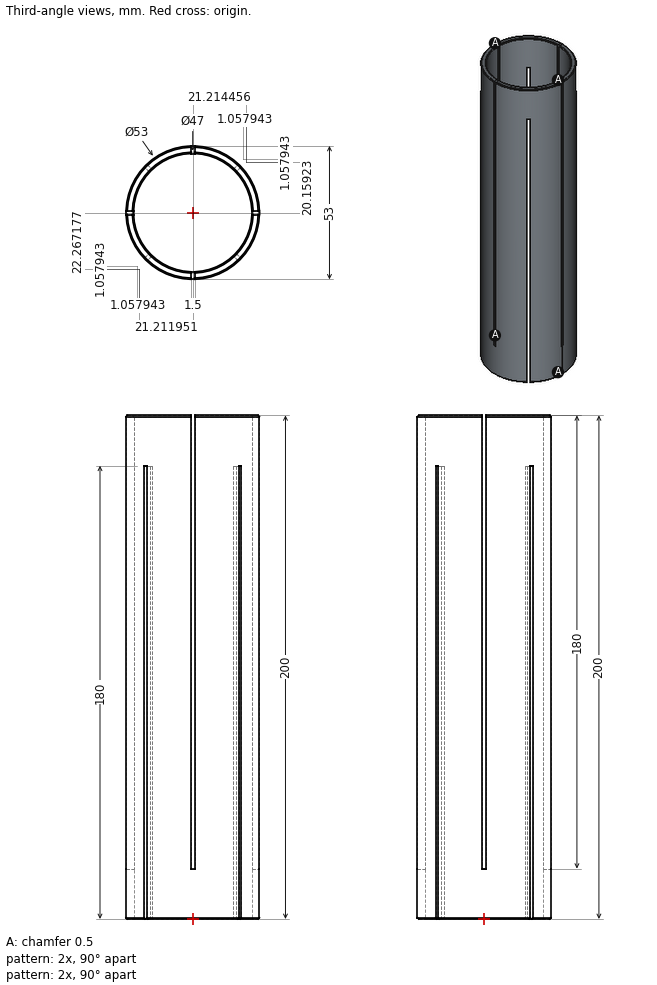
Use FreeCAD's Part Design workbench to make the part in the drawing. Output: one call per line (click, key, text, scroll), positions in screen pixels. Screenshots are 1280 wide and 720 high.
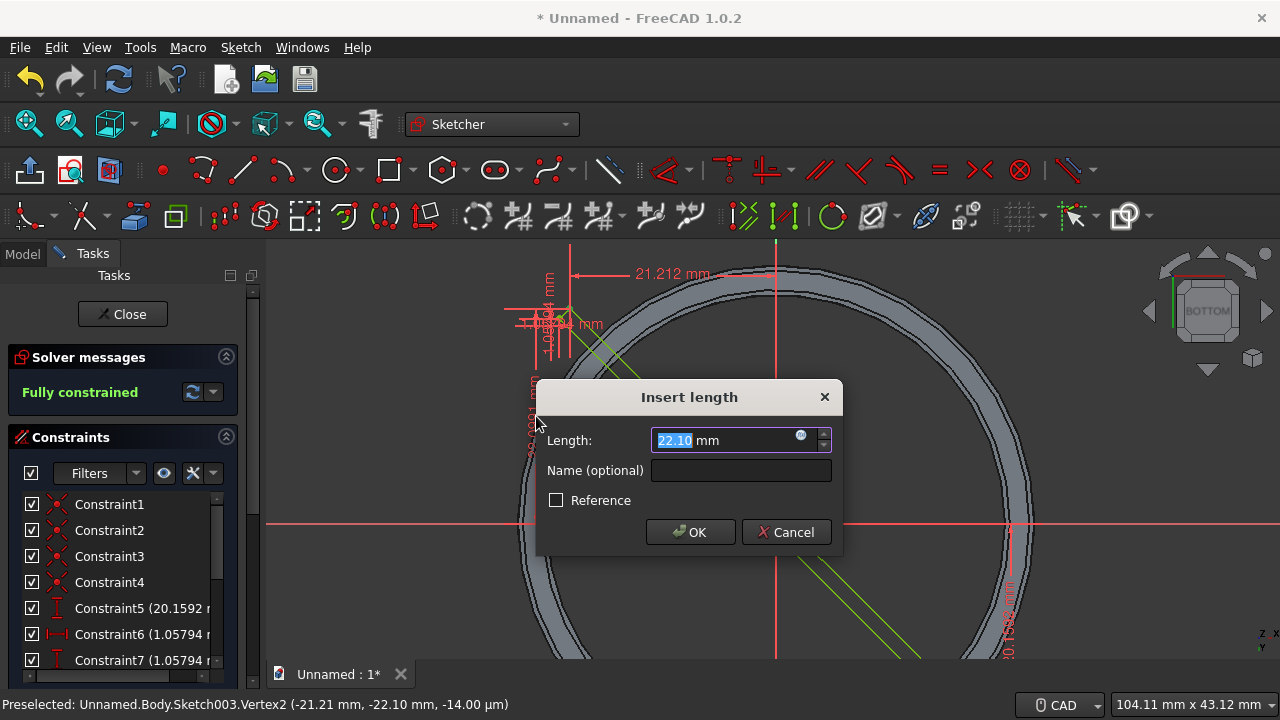
text(22.267177)
key(Return)
key(Escape)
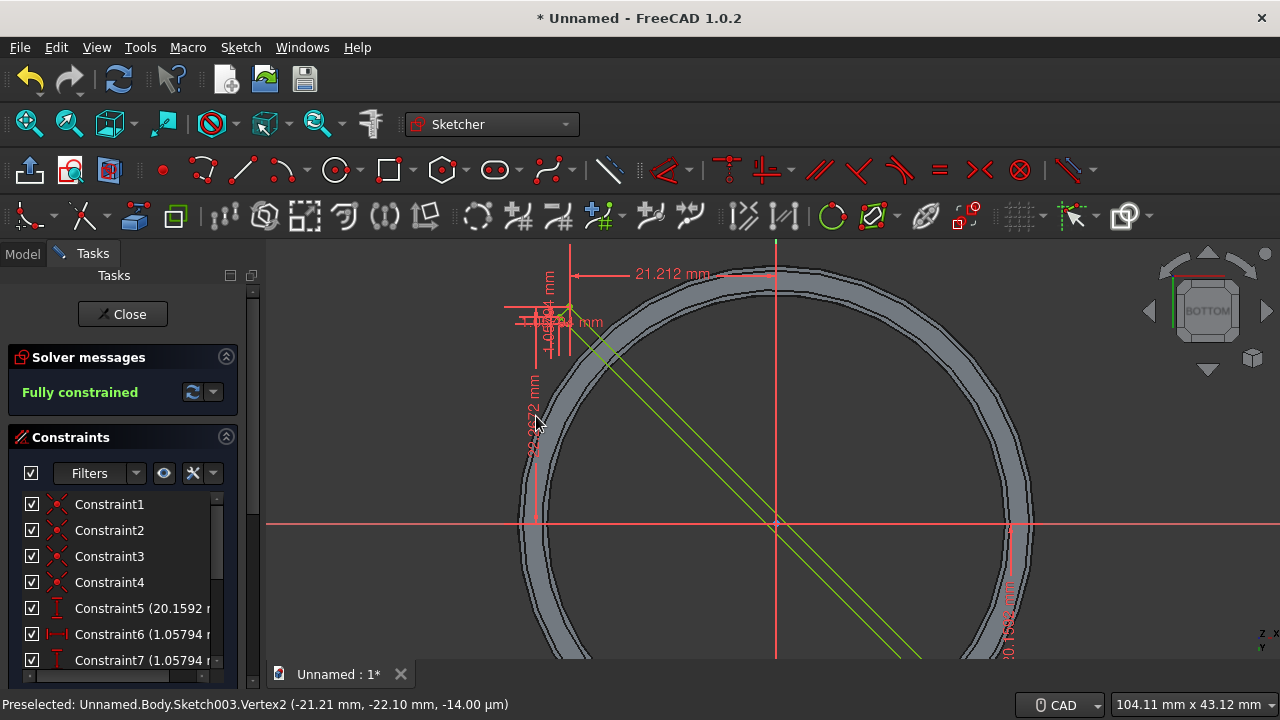
click(123, 314)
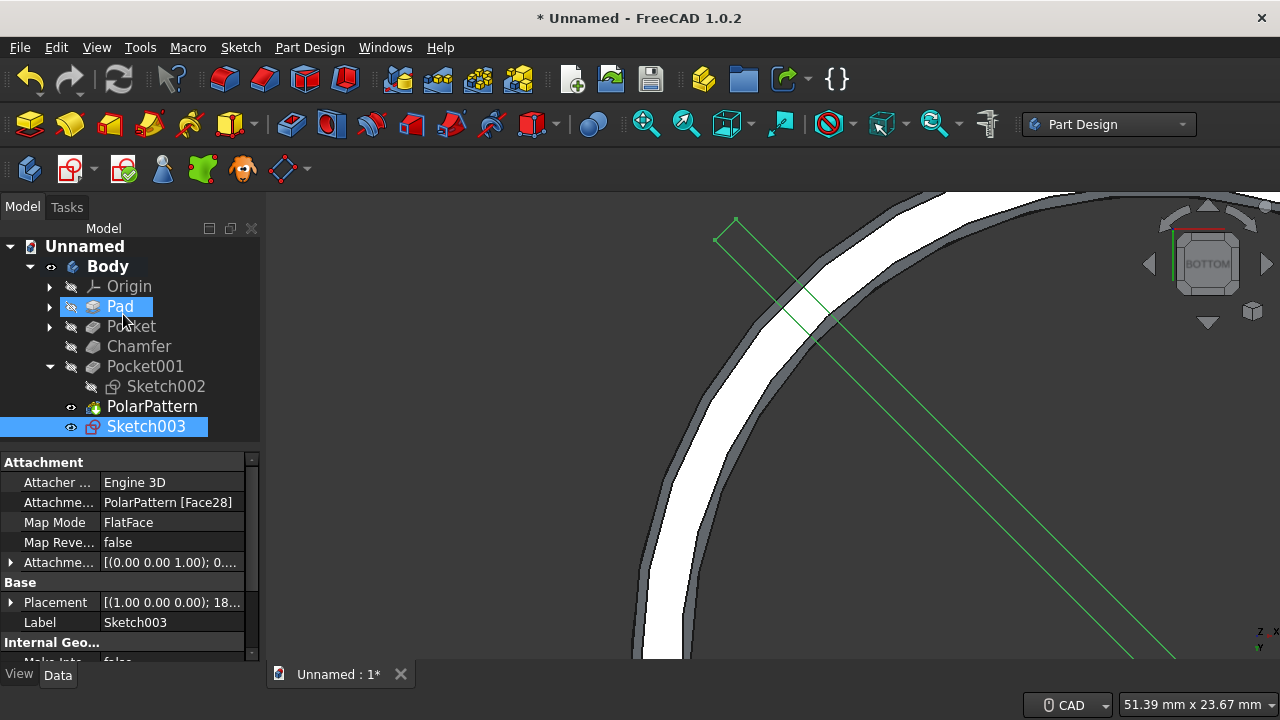
click(292, 124)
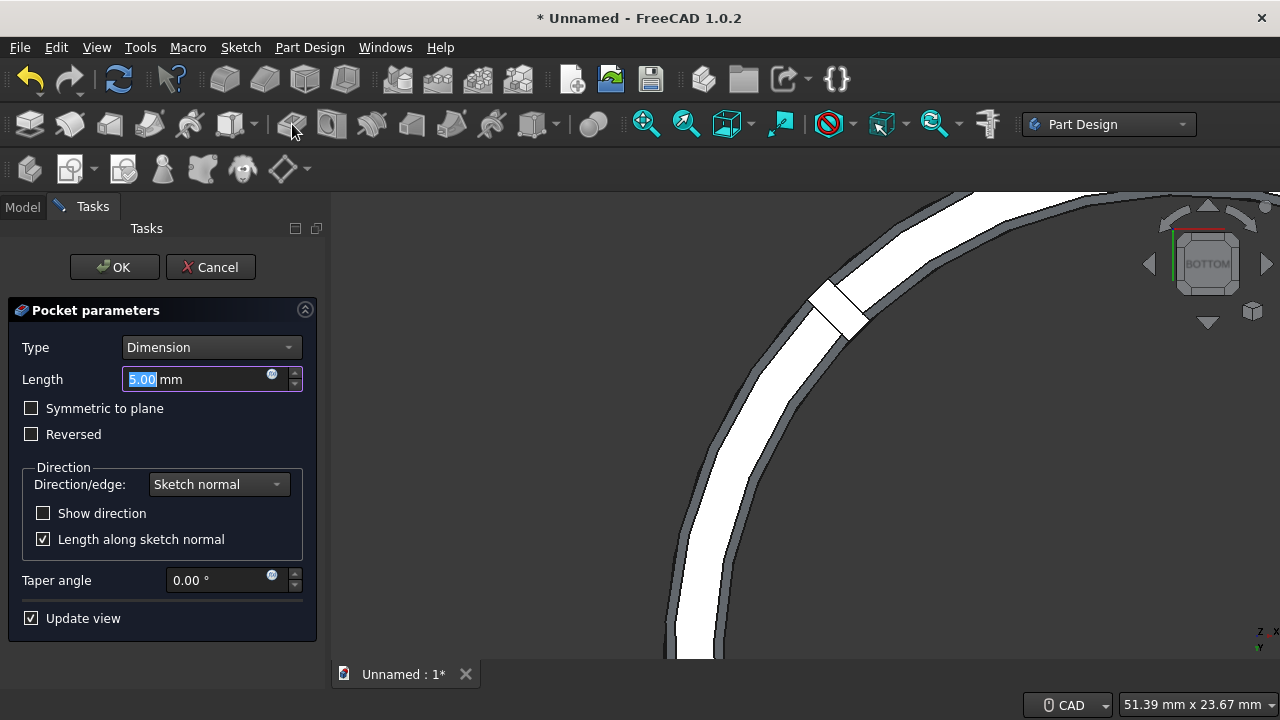
text(180)
key(Tab)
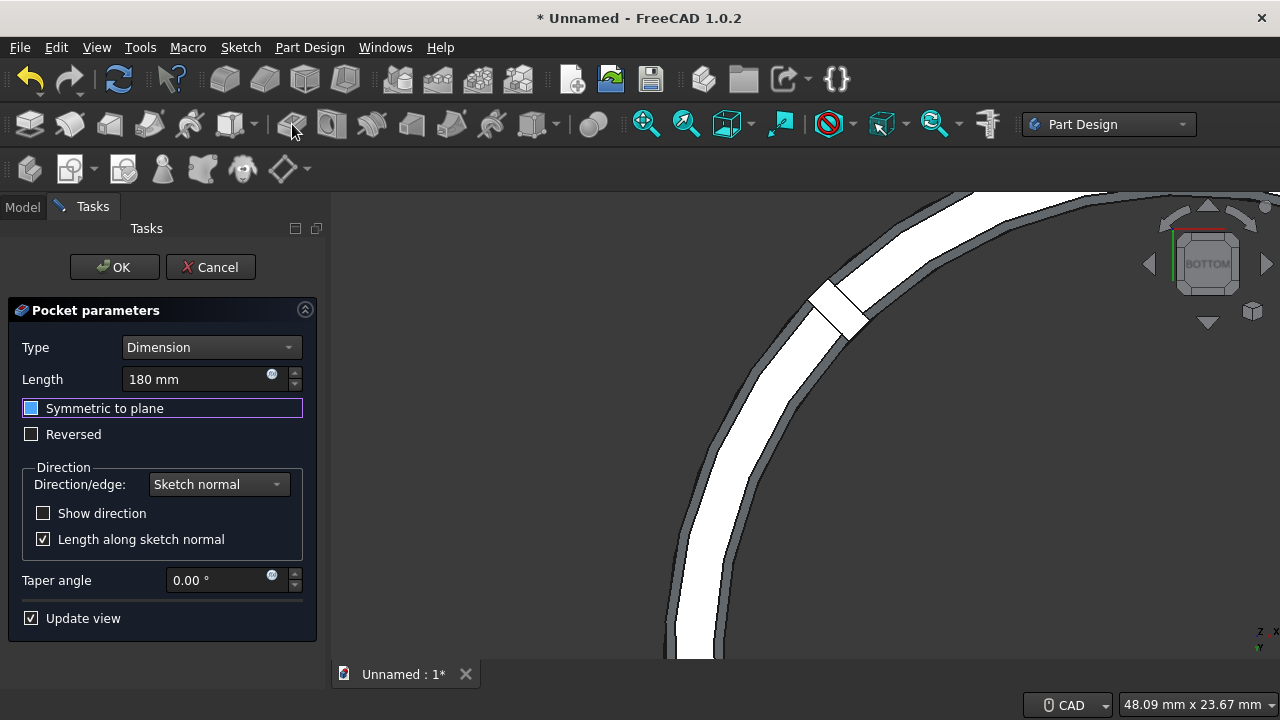
click(115, 267)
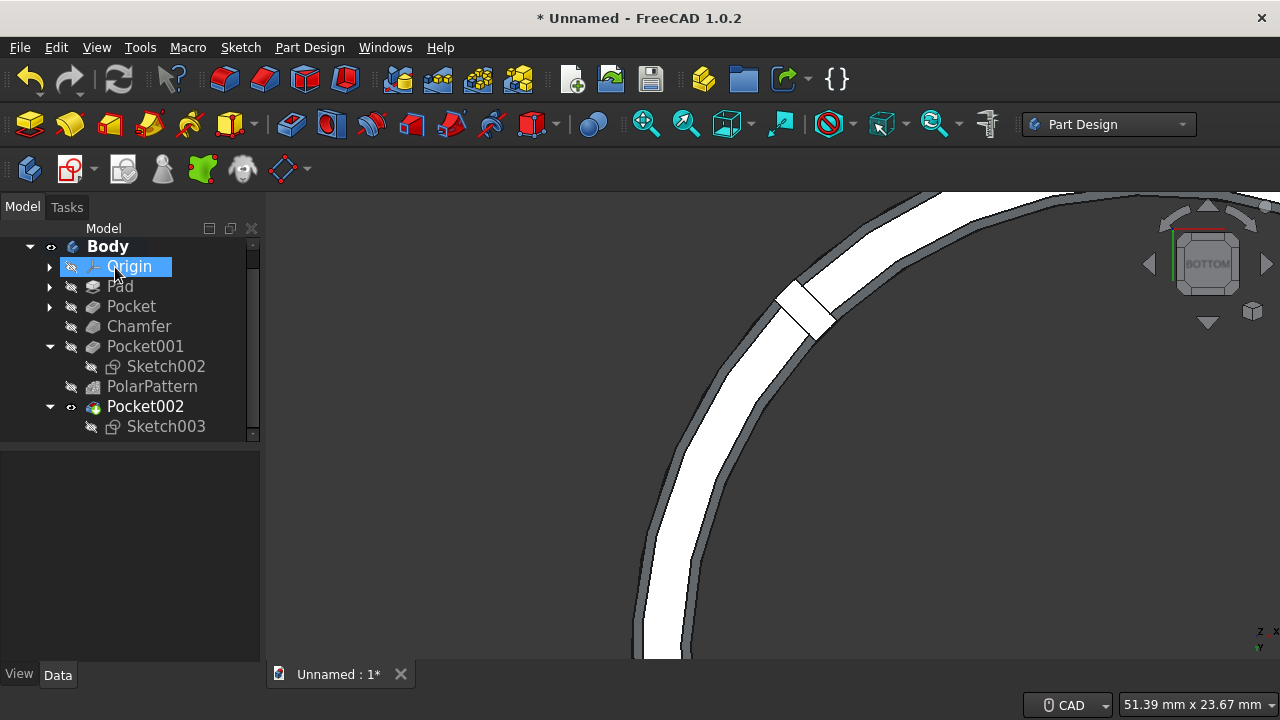
click(648, 124)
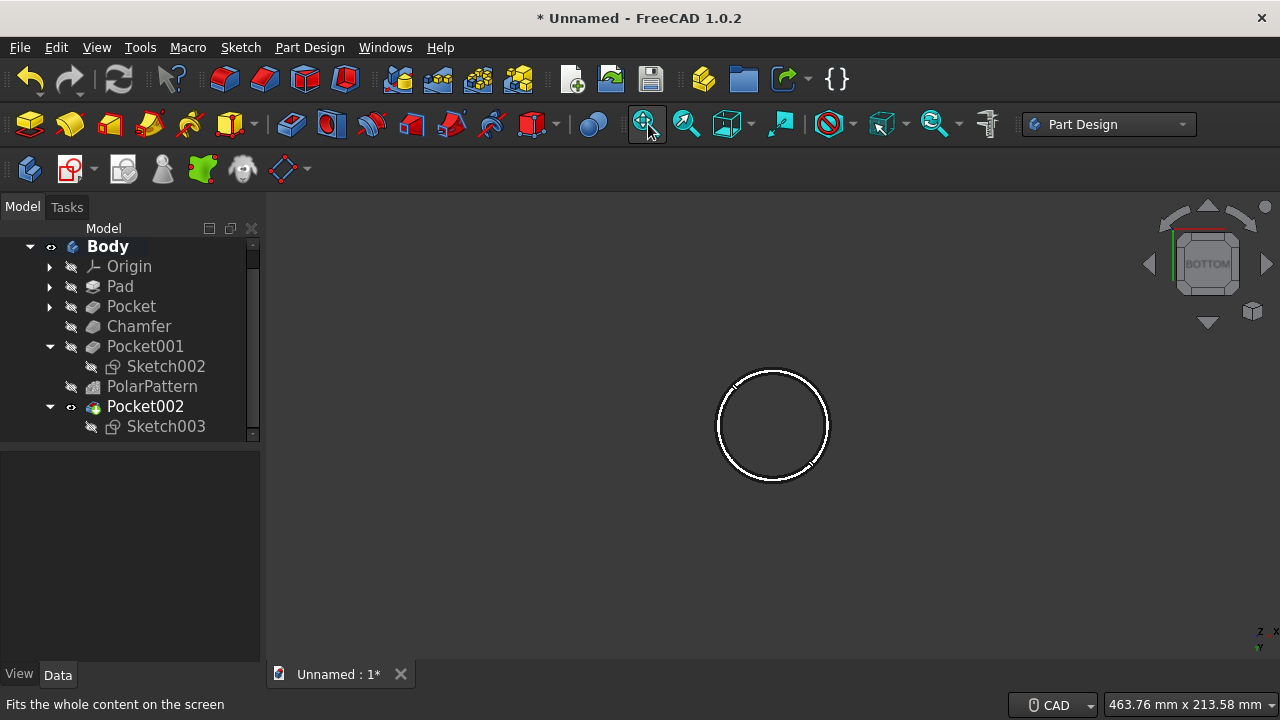
click(116, 407)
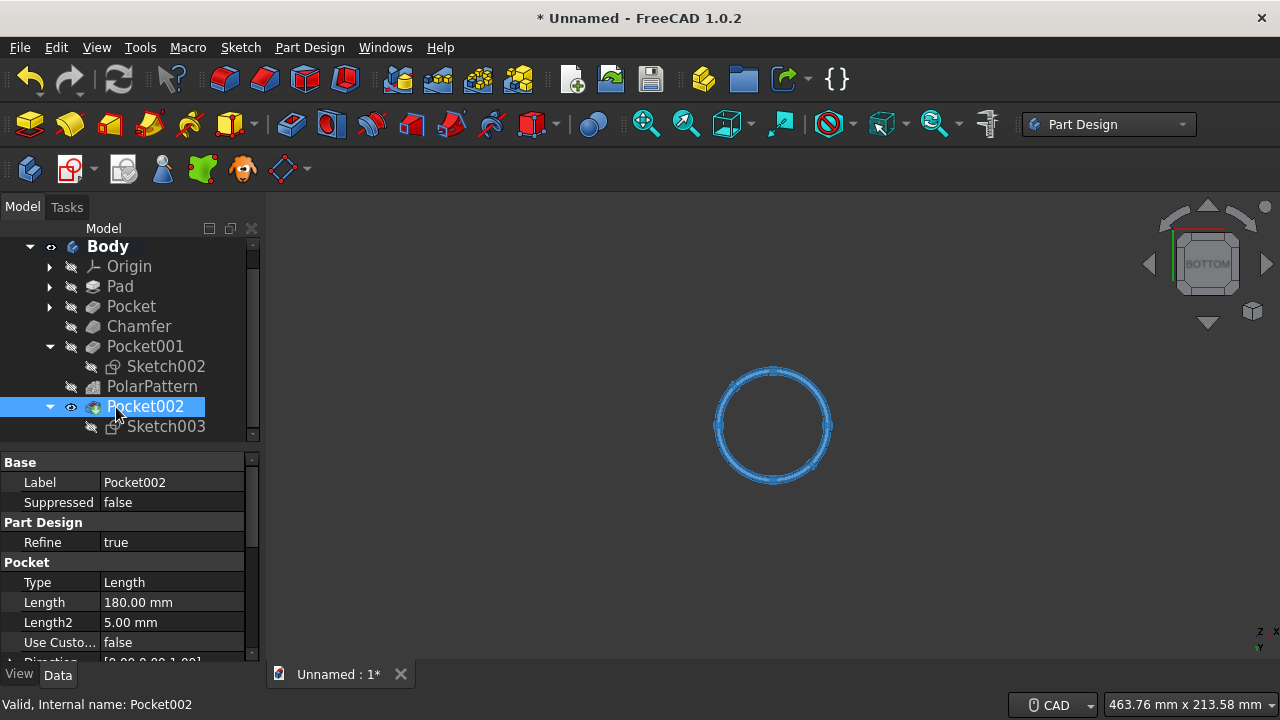
click(478, 80)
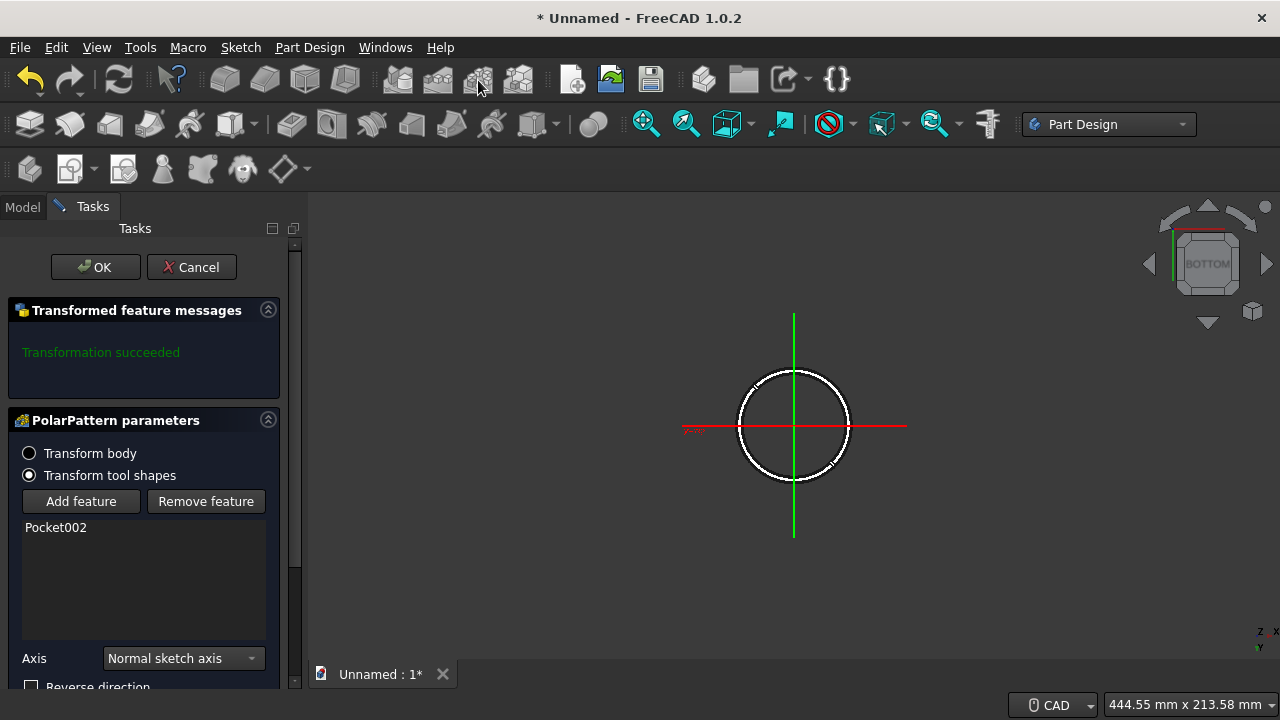
click(184, 658)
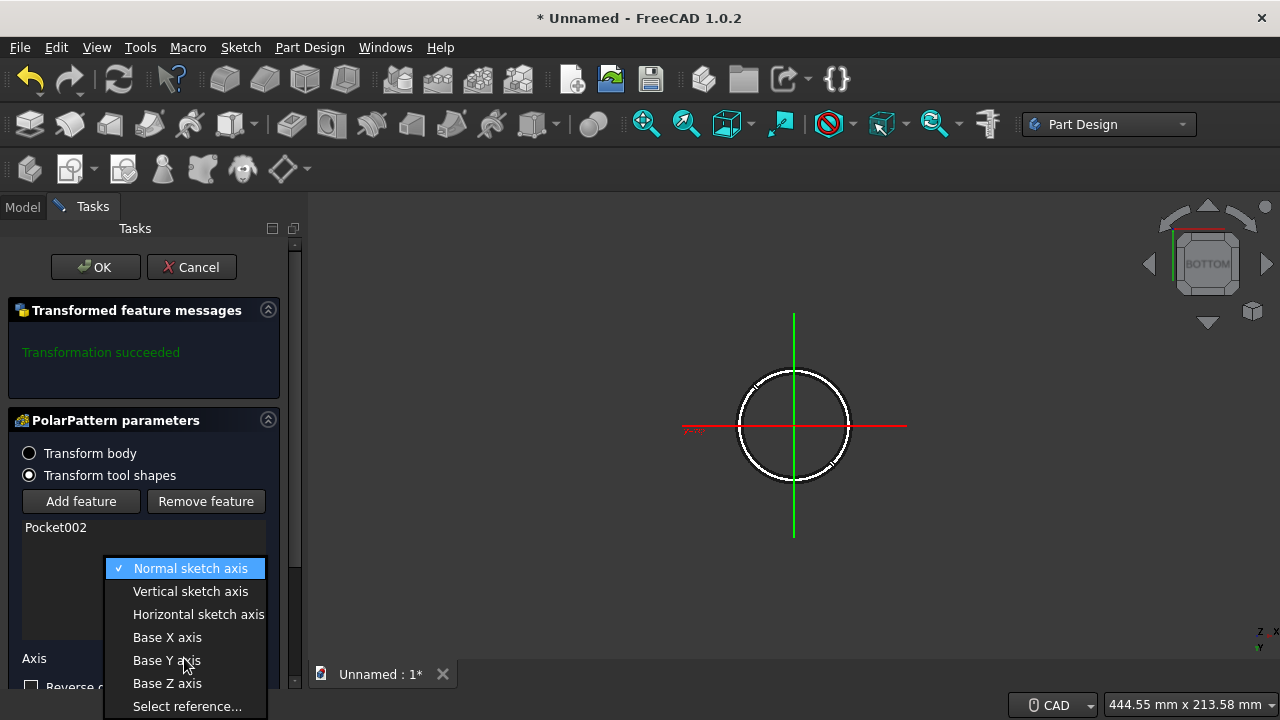
click(184, 684)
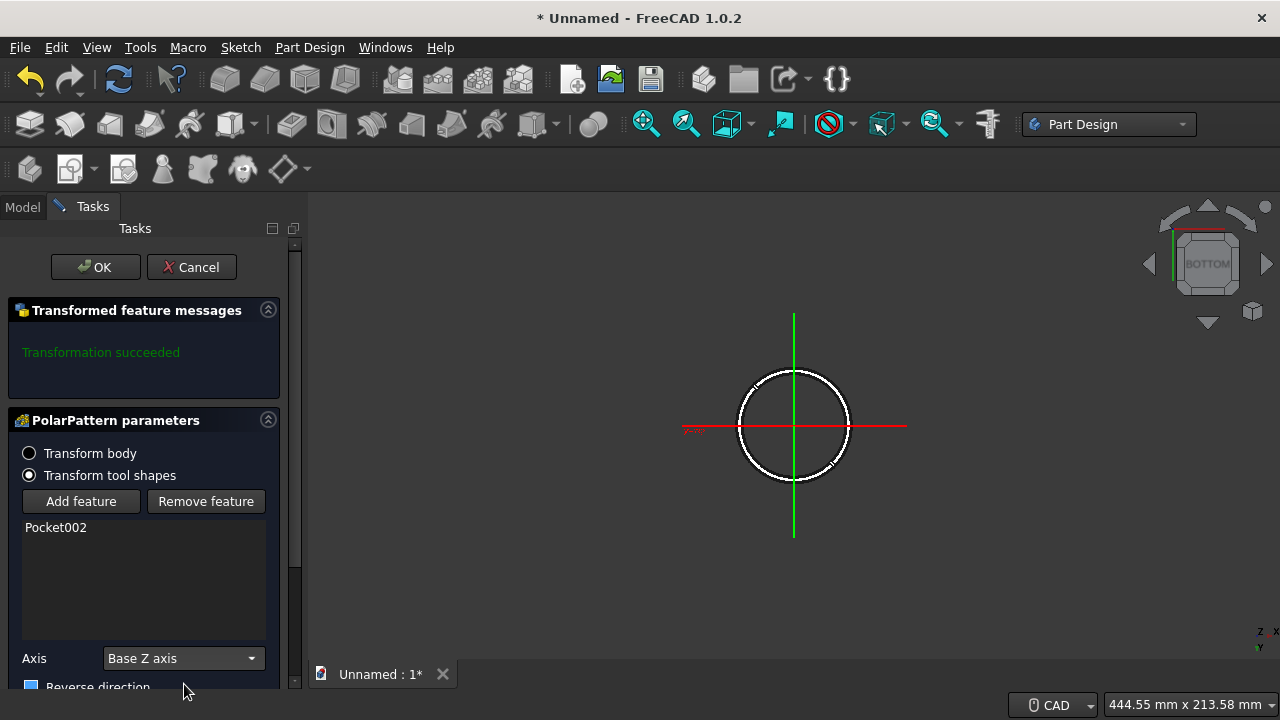
scroll(295, 463, down, 2)